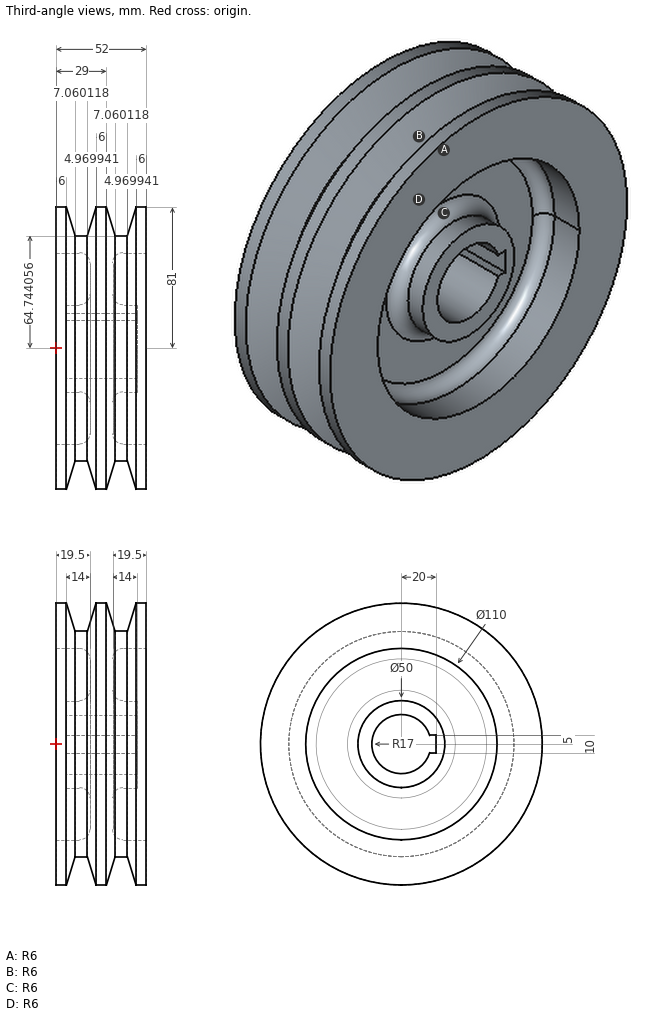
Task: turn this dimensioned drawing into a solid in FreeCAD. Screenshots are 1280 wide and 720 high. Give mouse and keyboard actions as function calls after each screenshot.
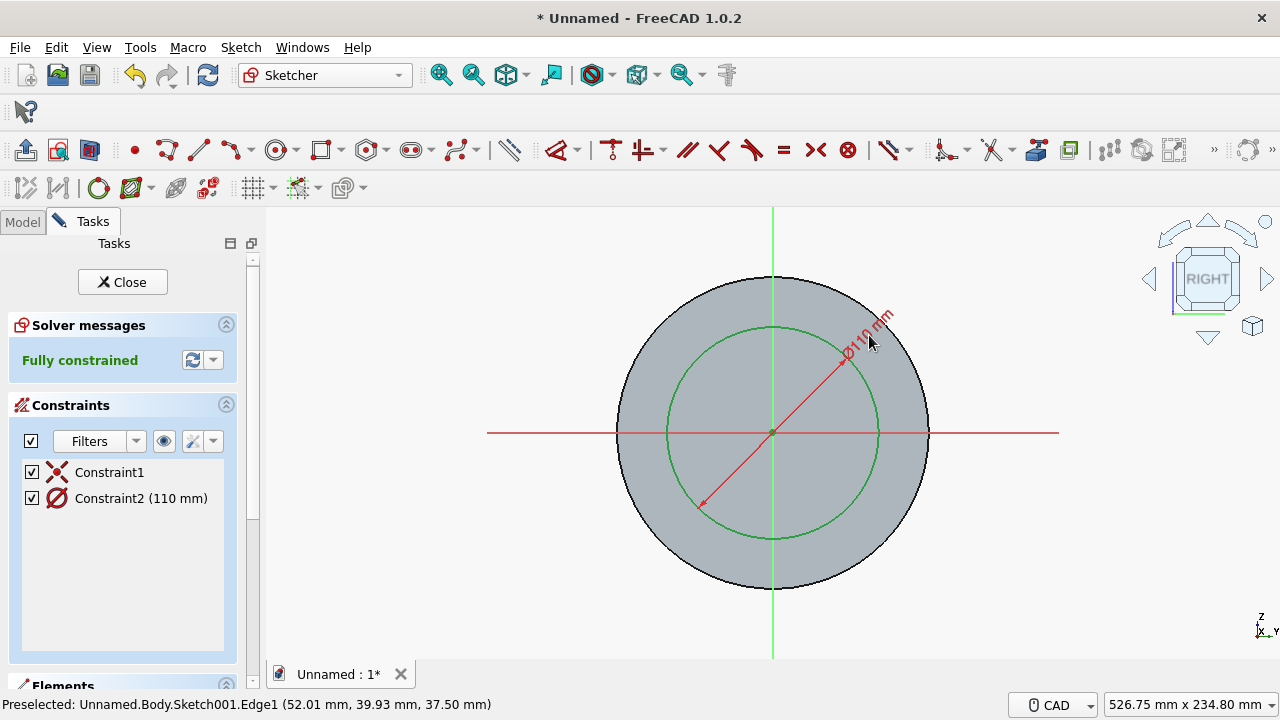
click(123, 282)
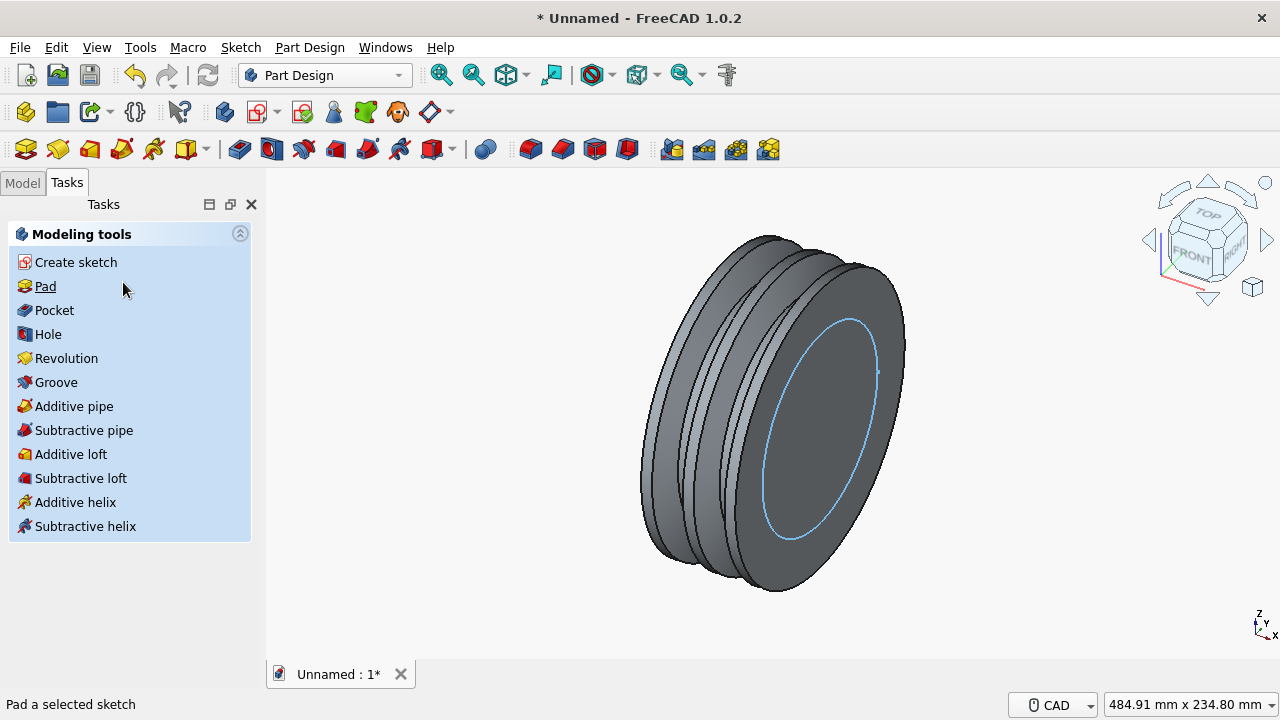
click(240, 150)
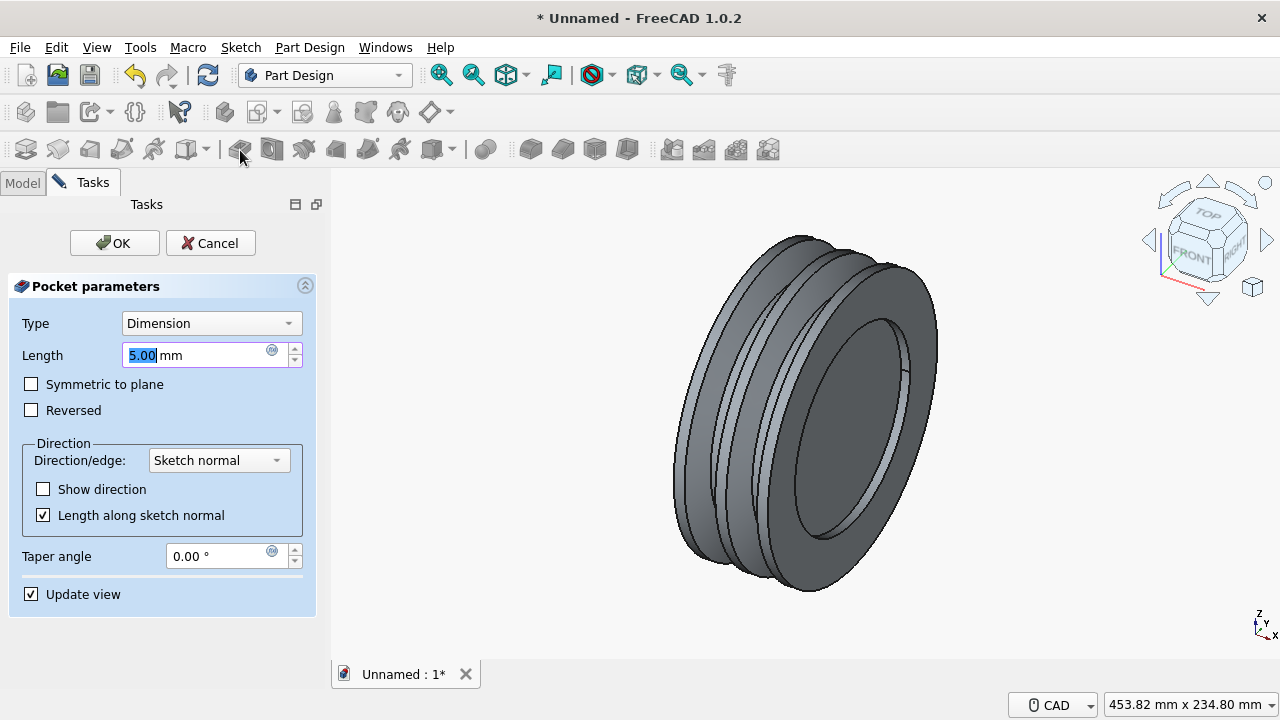
text(19.5)
key(Tab)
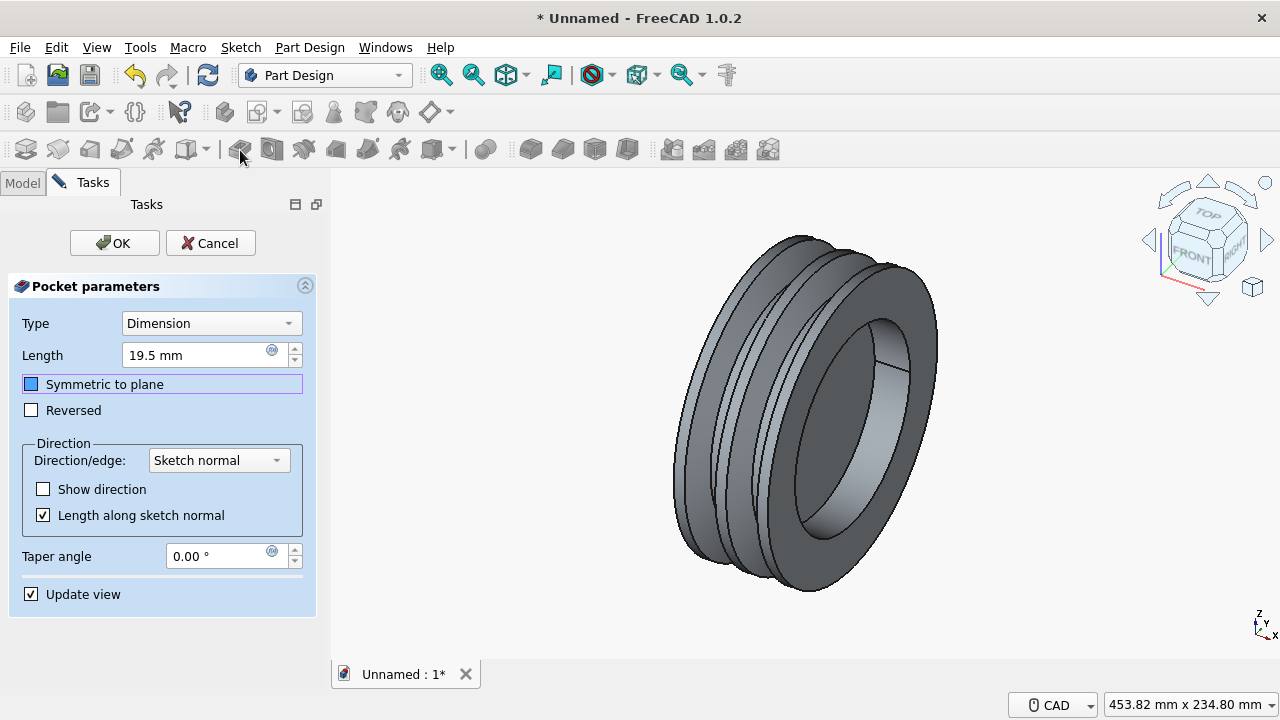
click(115, 243)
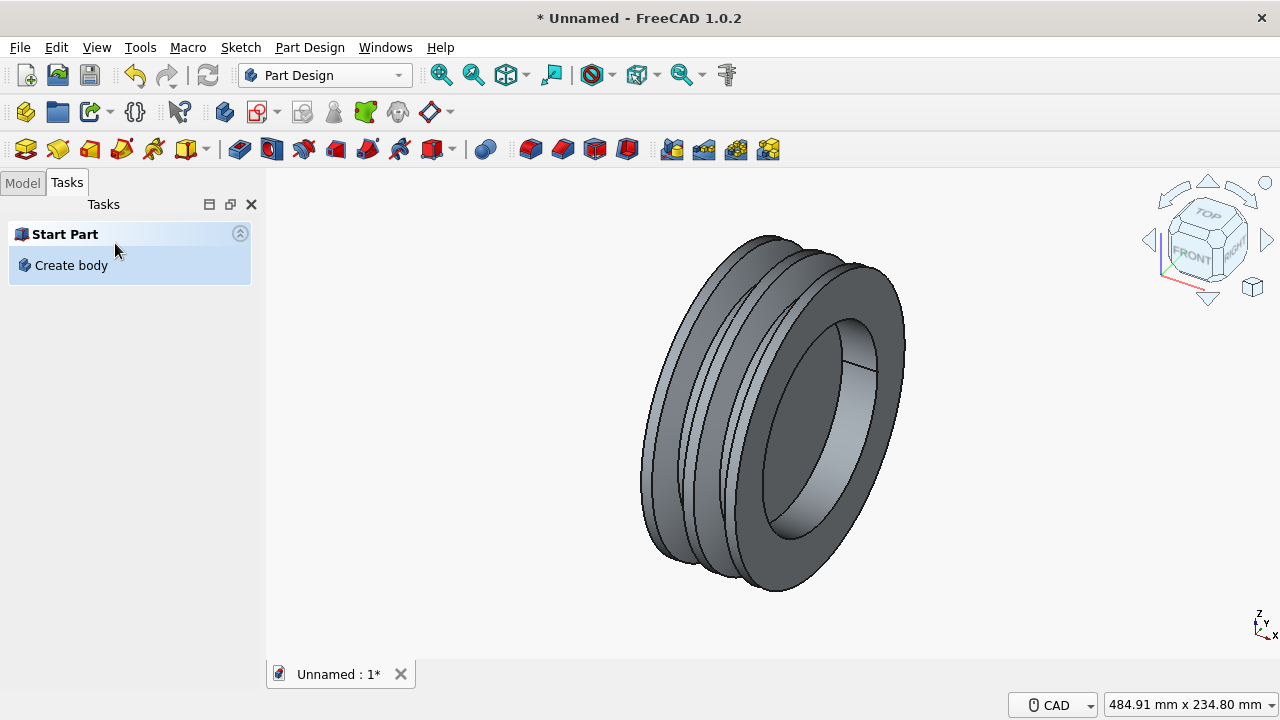
click(23, 182)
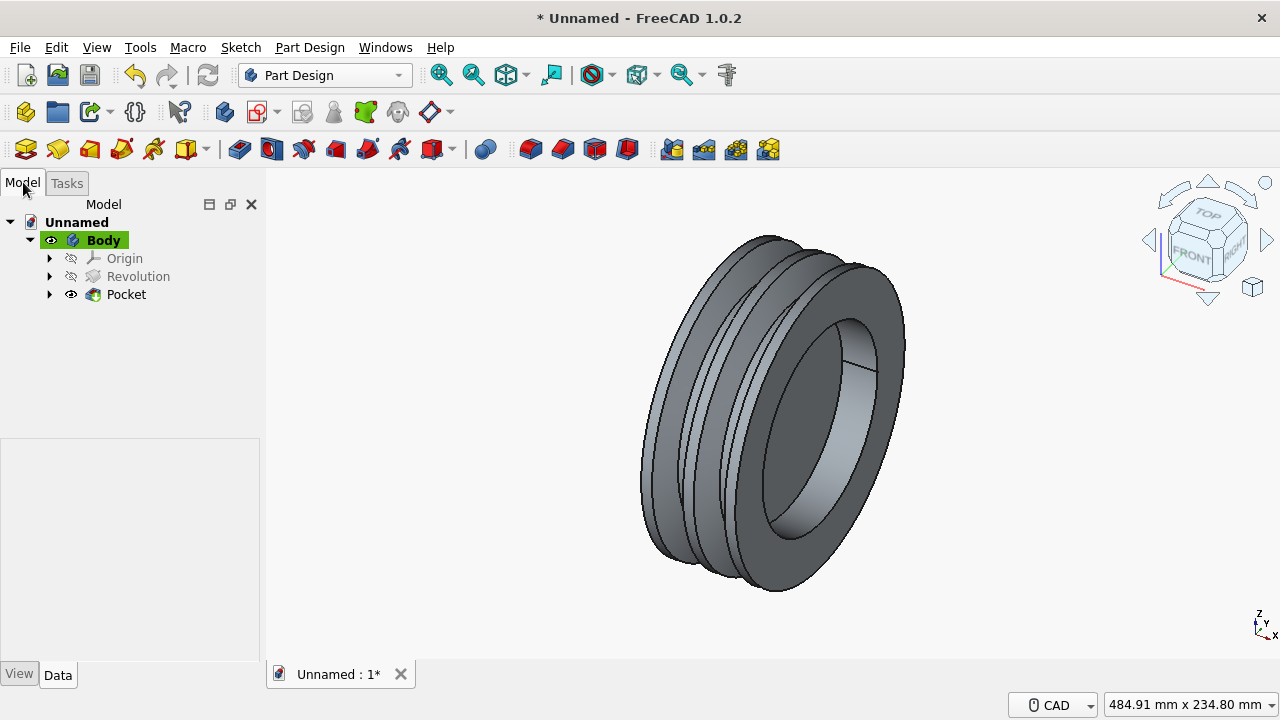
click(50, 258)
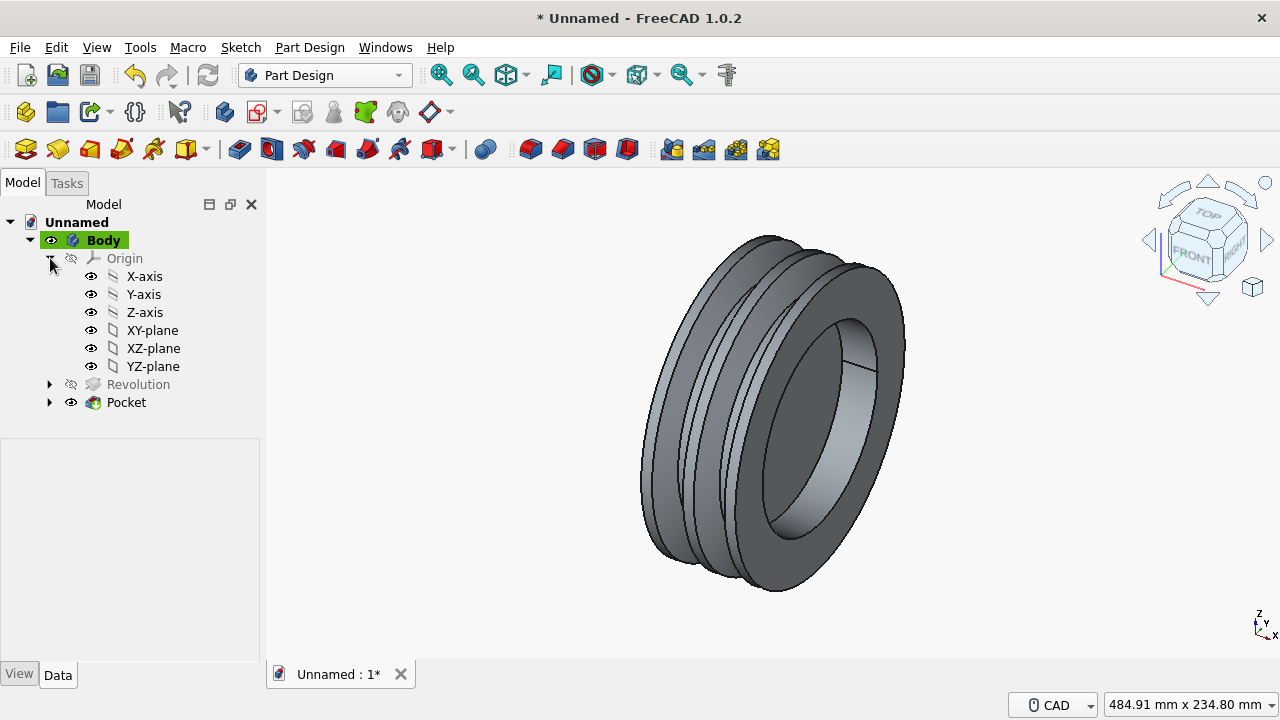
click(136, 366)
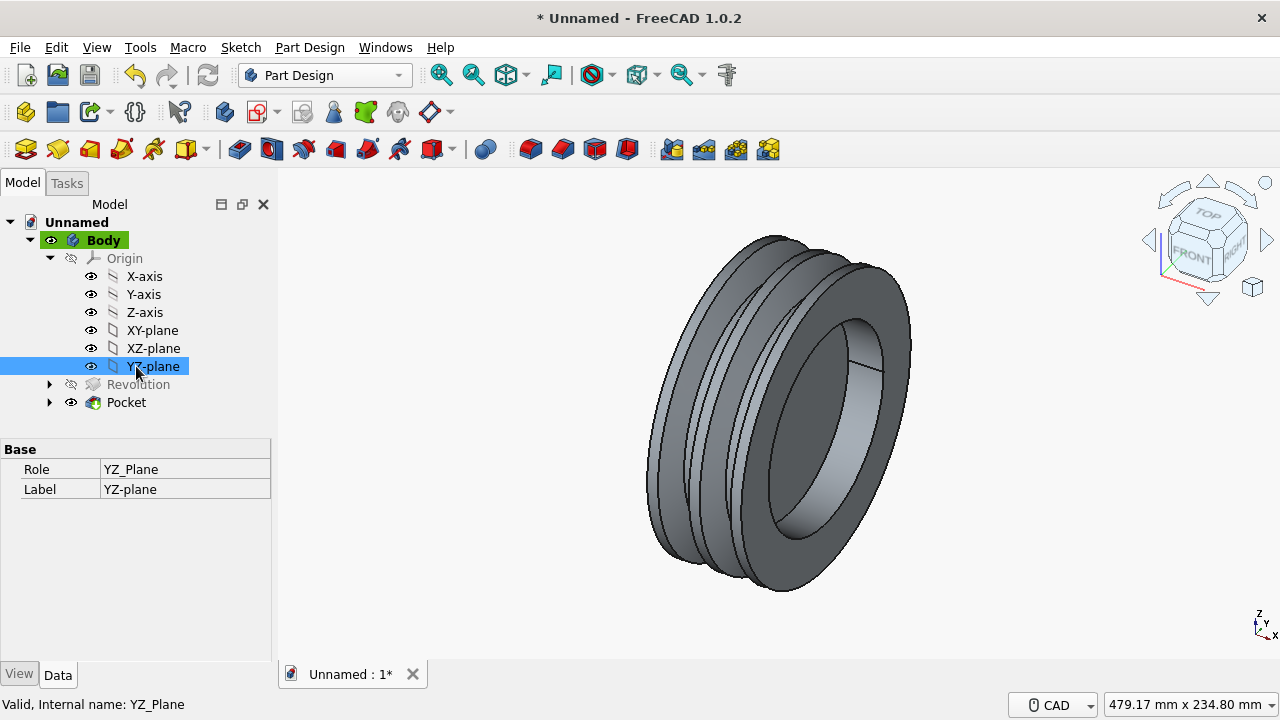
click(430, 112)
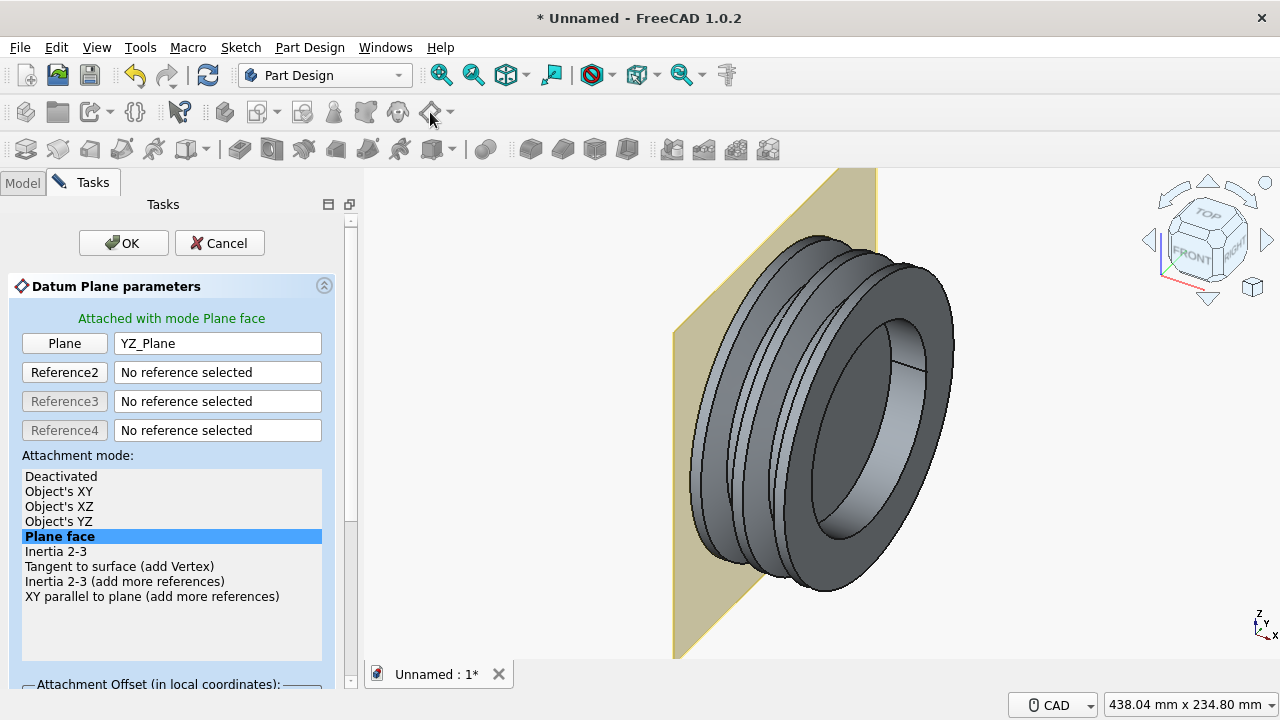
scroll(351, 451, down, 3)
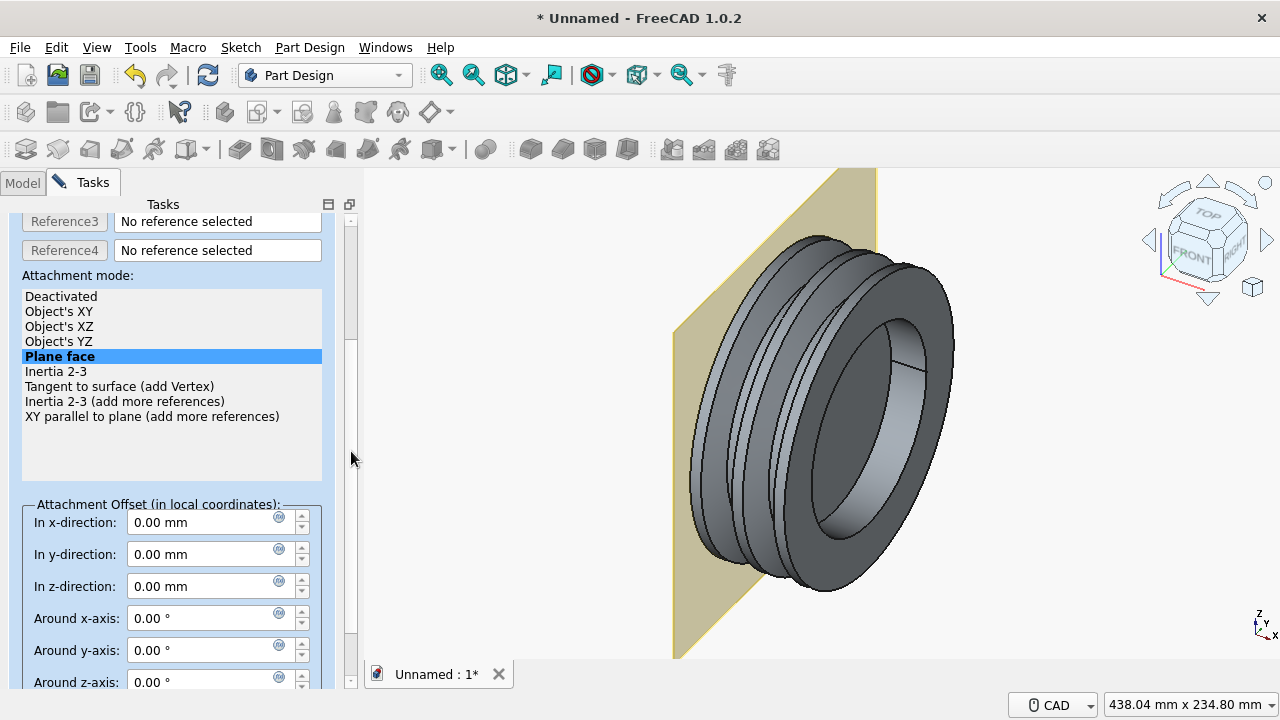
triple_click(210, 586)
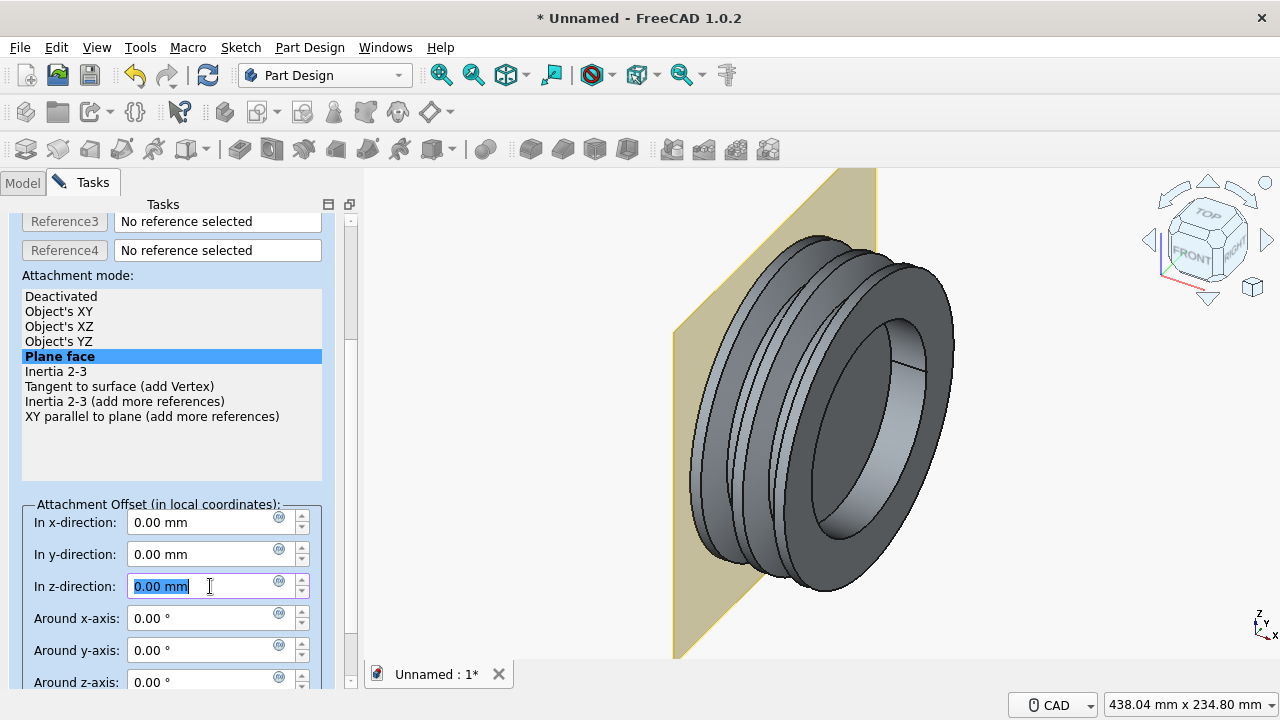
text(19.5)
key(Tab)